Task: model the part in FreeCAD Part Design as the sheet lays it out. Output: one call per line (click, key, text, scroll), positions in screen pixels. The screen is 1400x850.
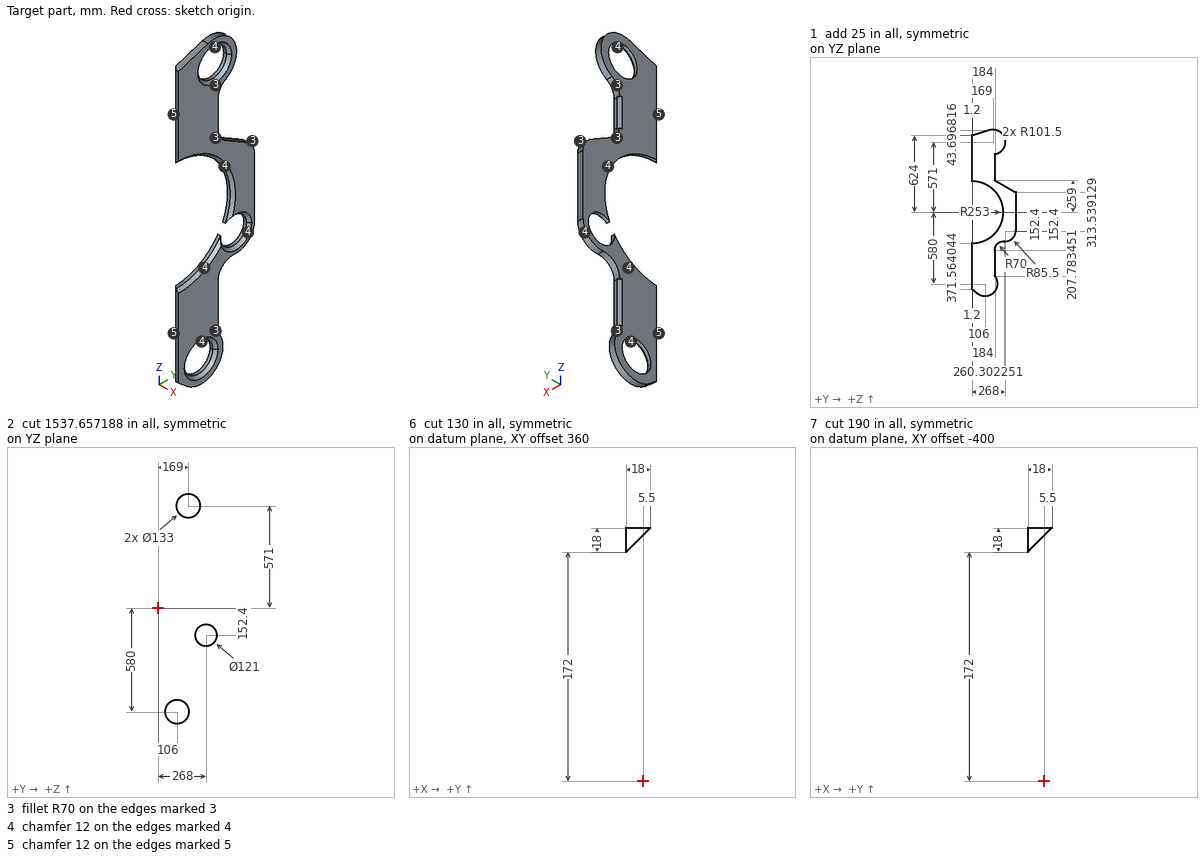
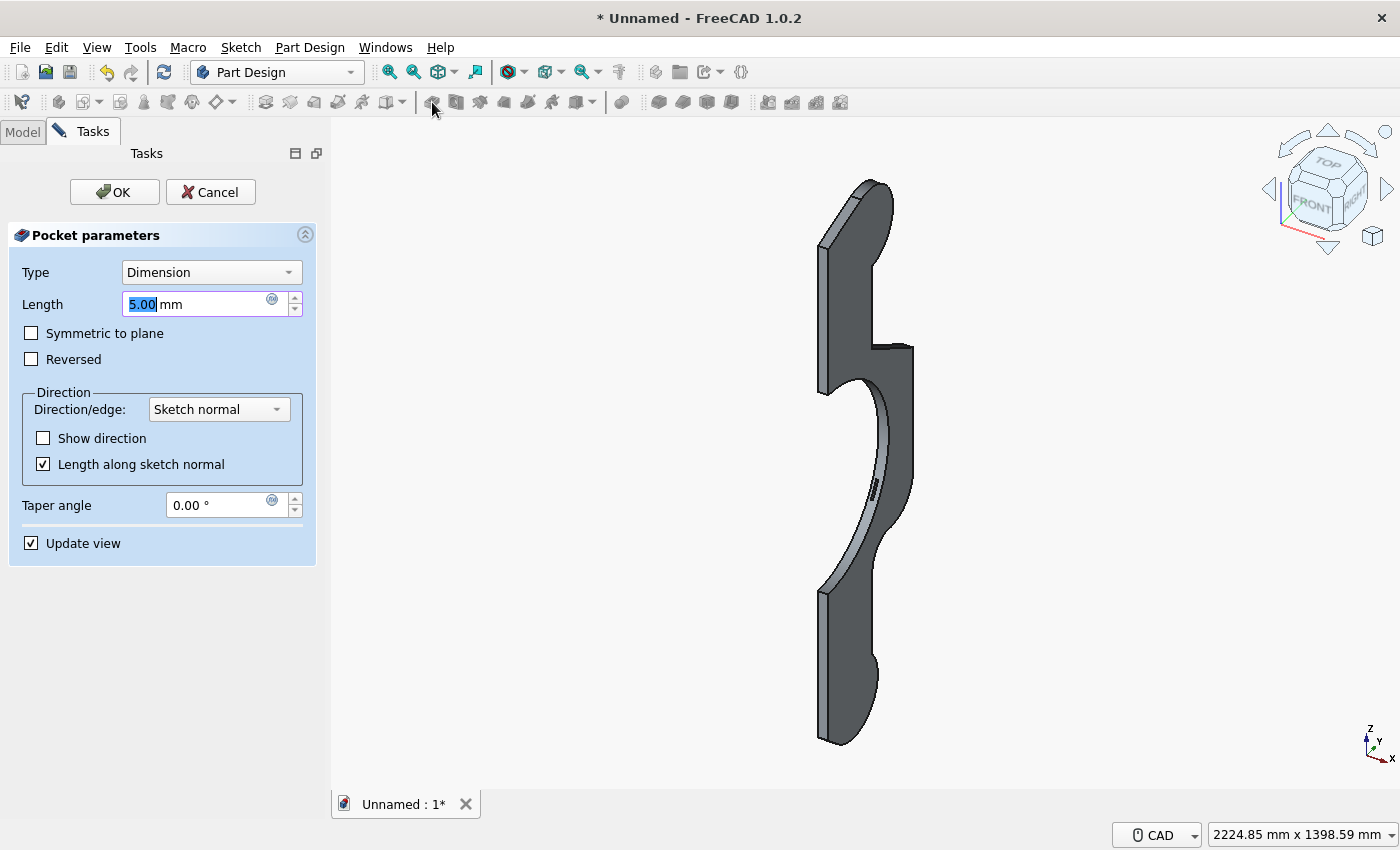
text(1537.657188)
key(Tab)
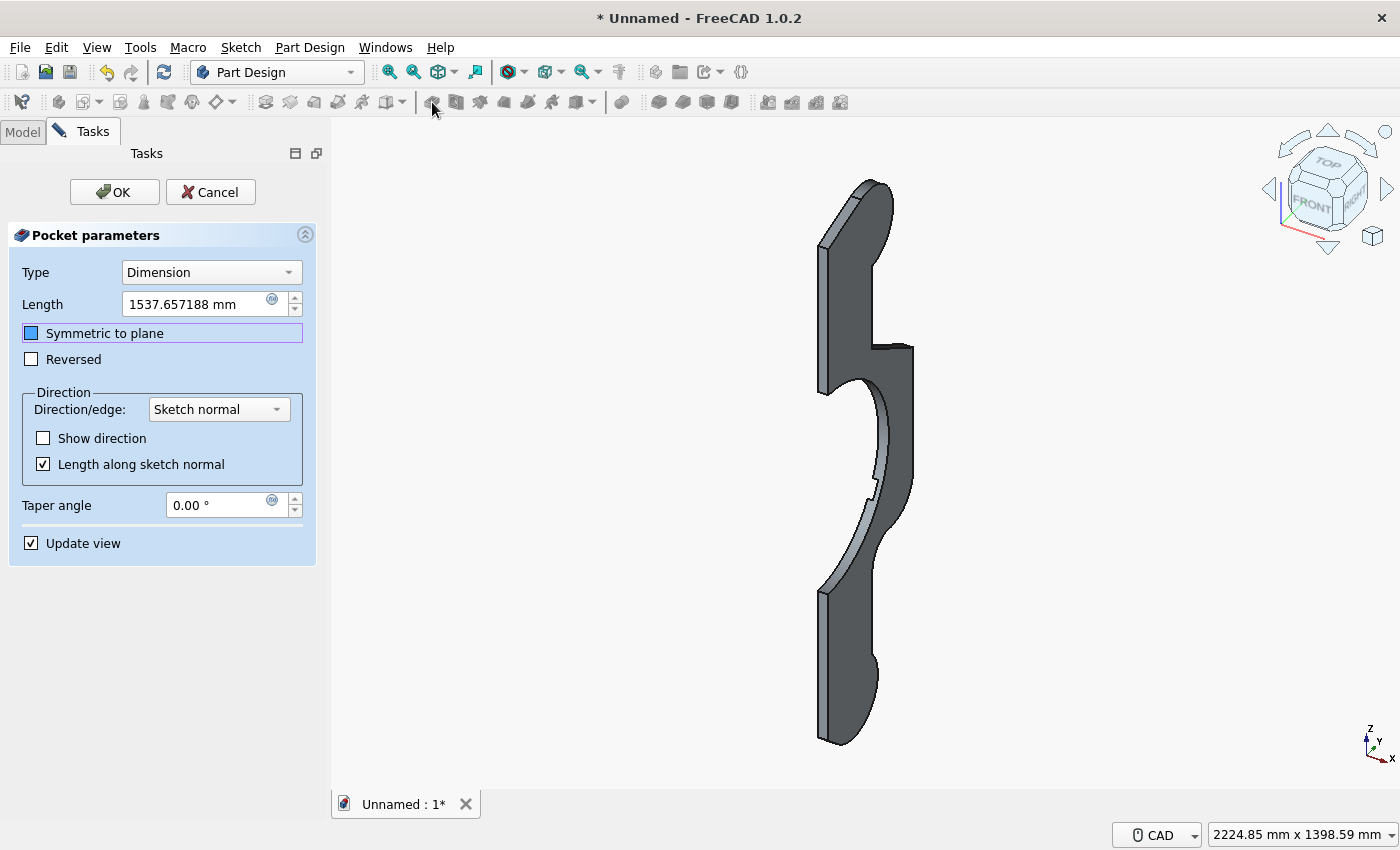
click(30, 333)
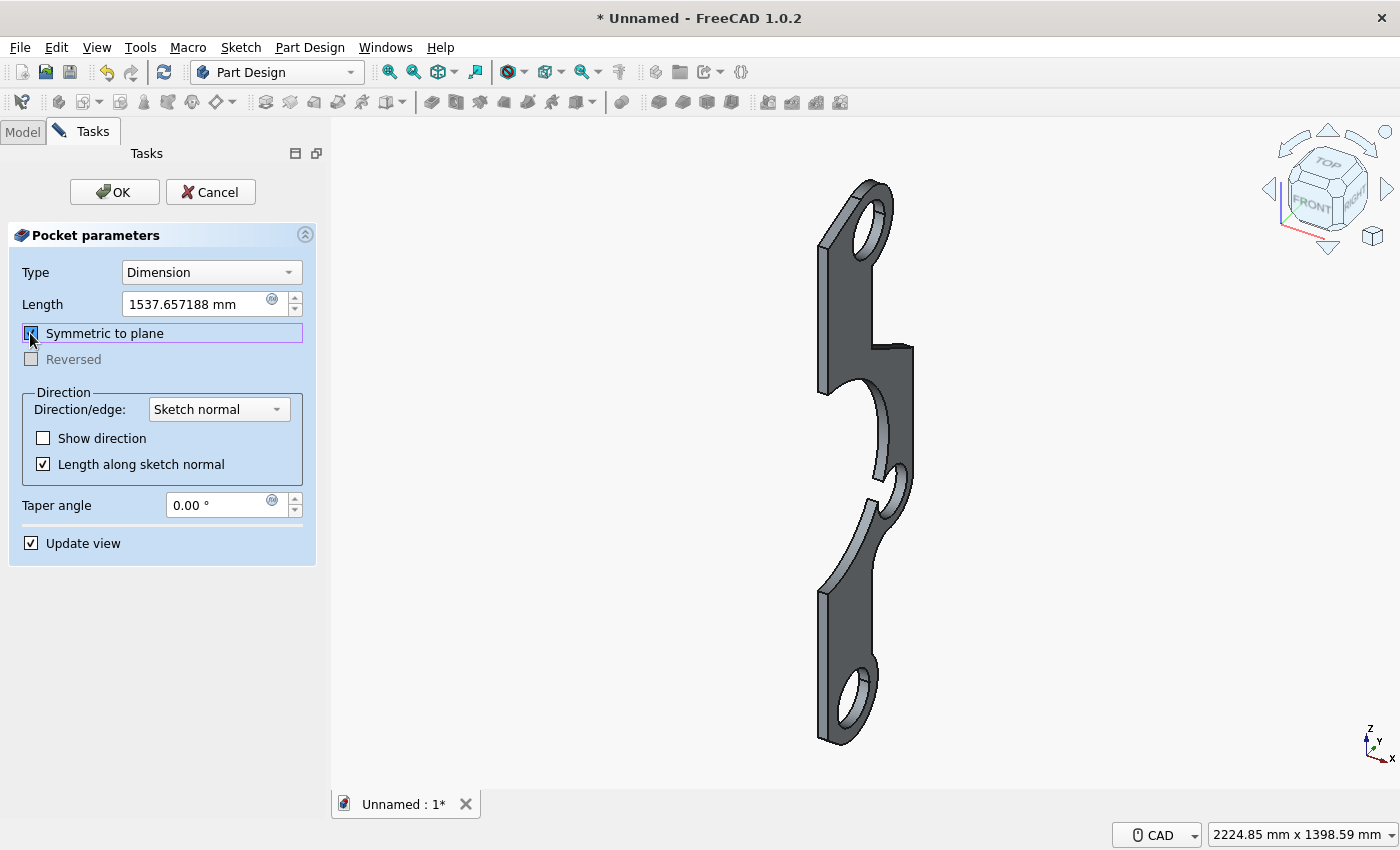
click(115, 192)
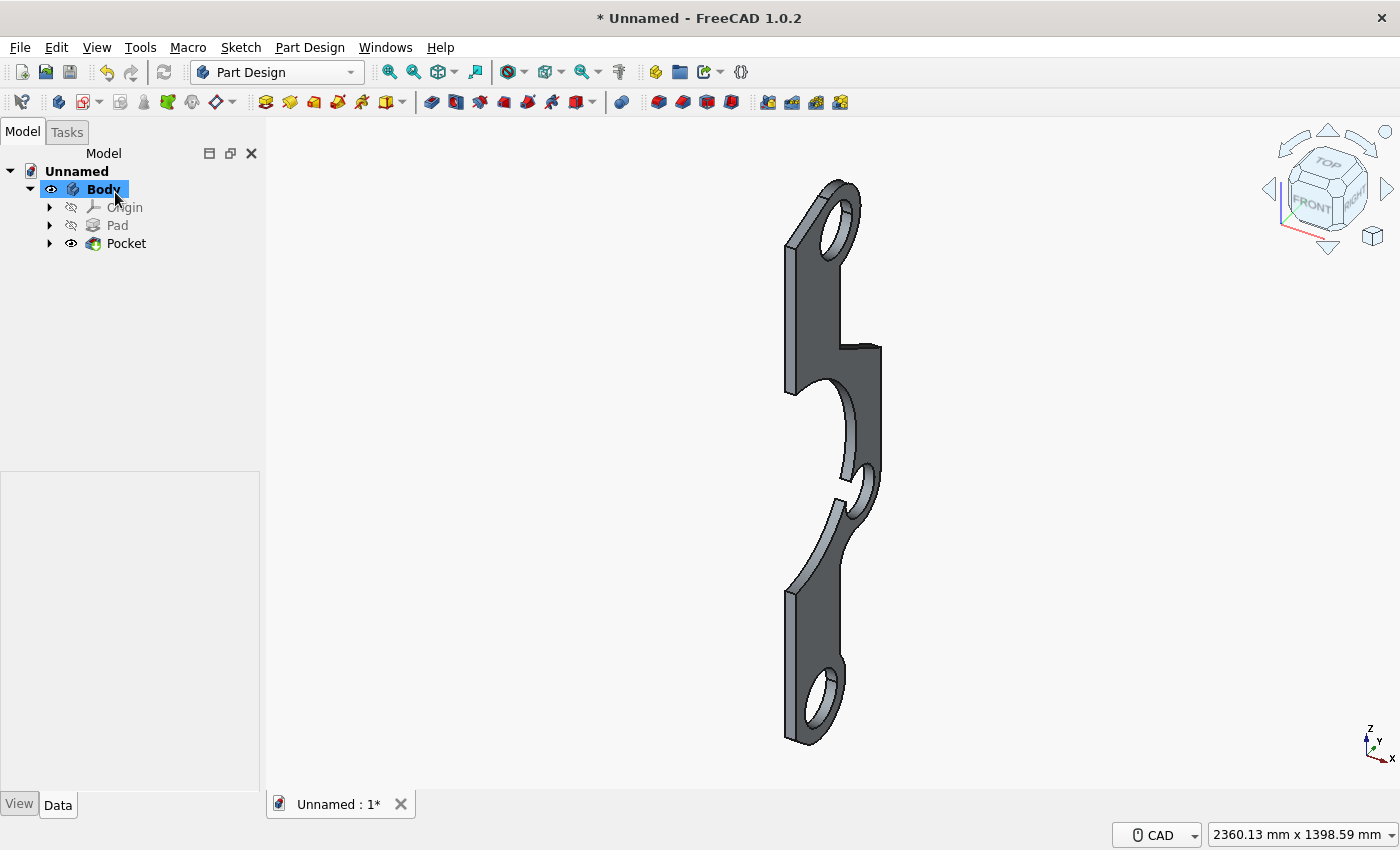
scroll(835, 263, up, 7)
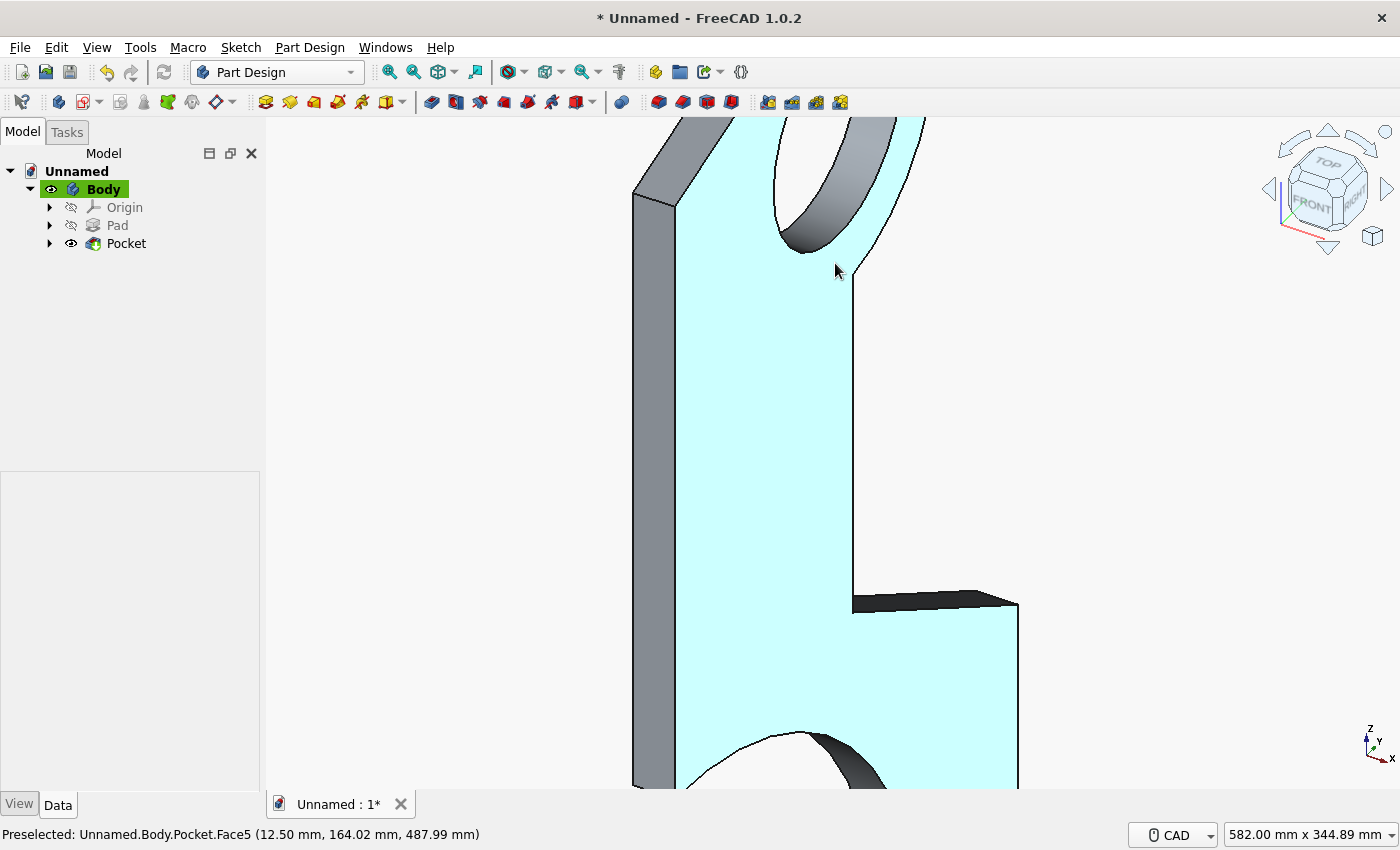
click(390, 72)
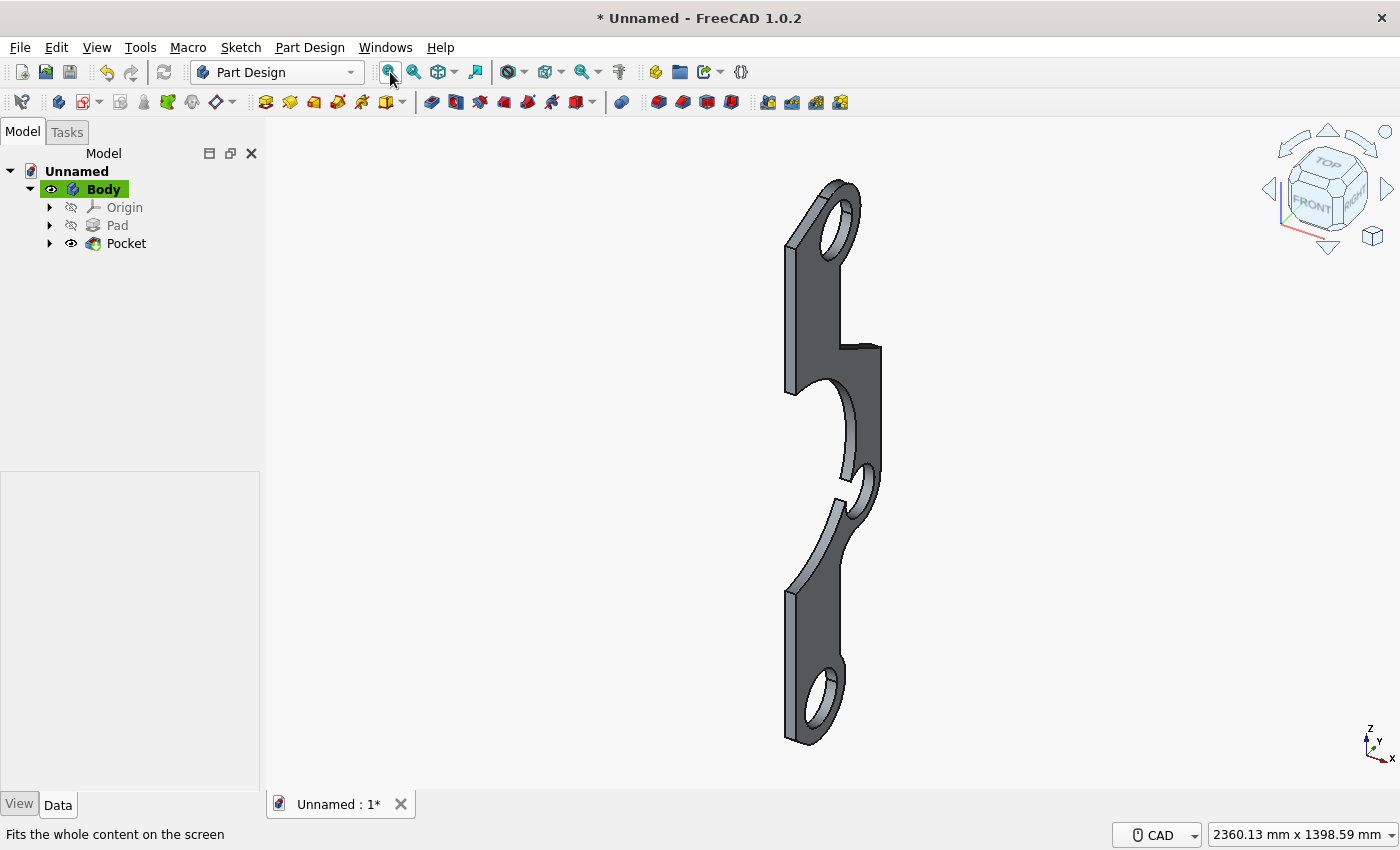
key(0)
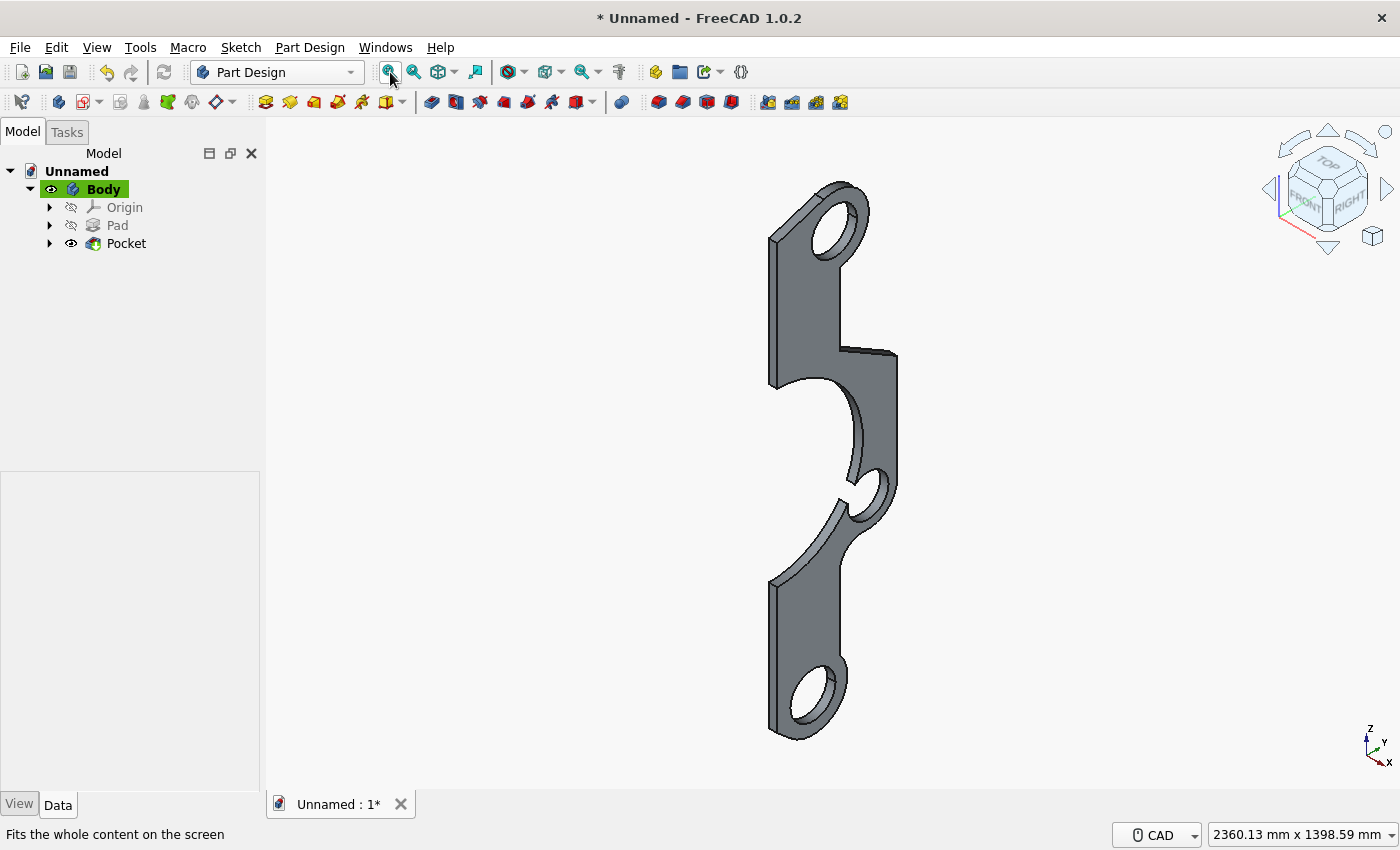
scroll(835, 264, up, 7)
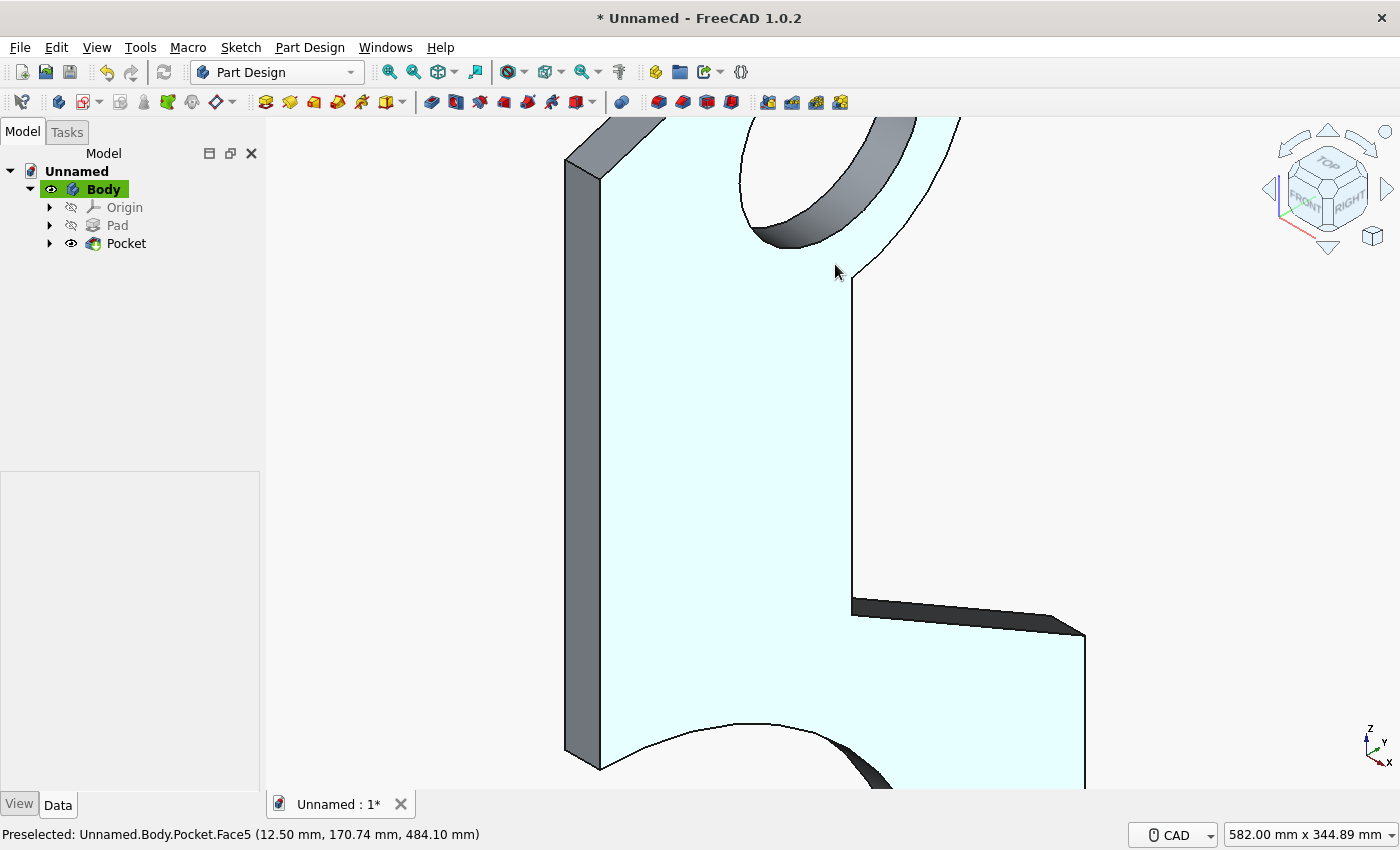
key(v)
key(f)